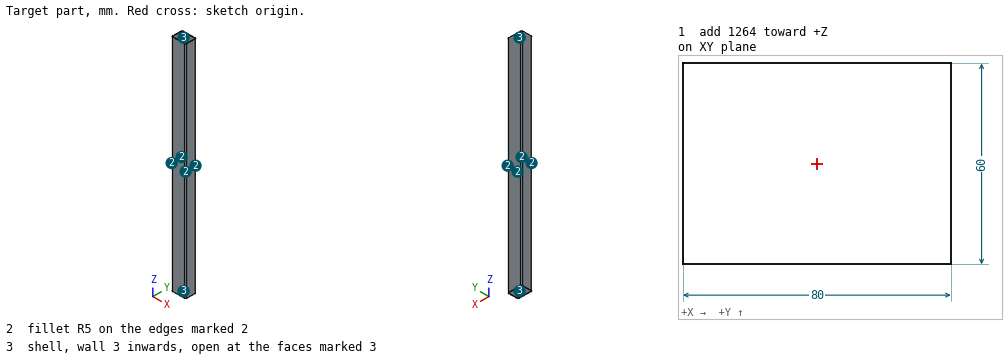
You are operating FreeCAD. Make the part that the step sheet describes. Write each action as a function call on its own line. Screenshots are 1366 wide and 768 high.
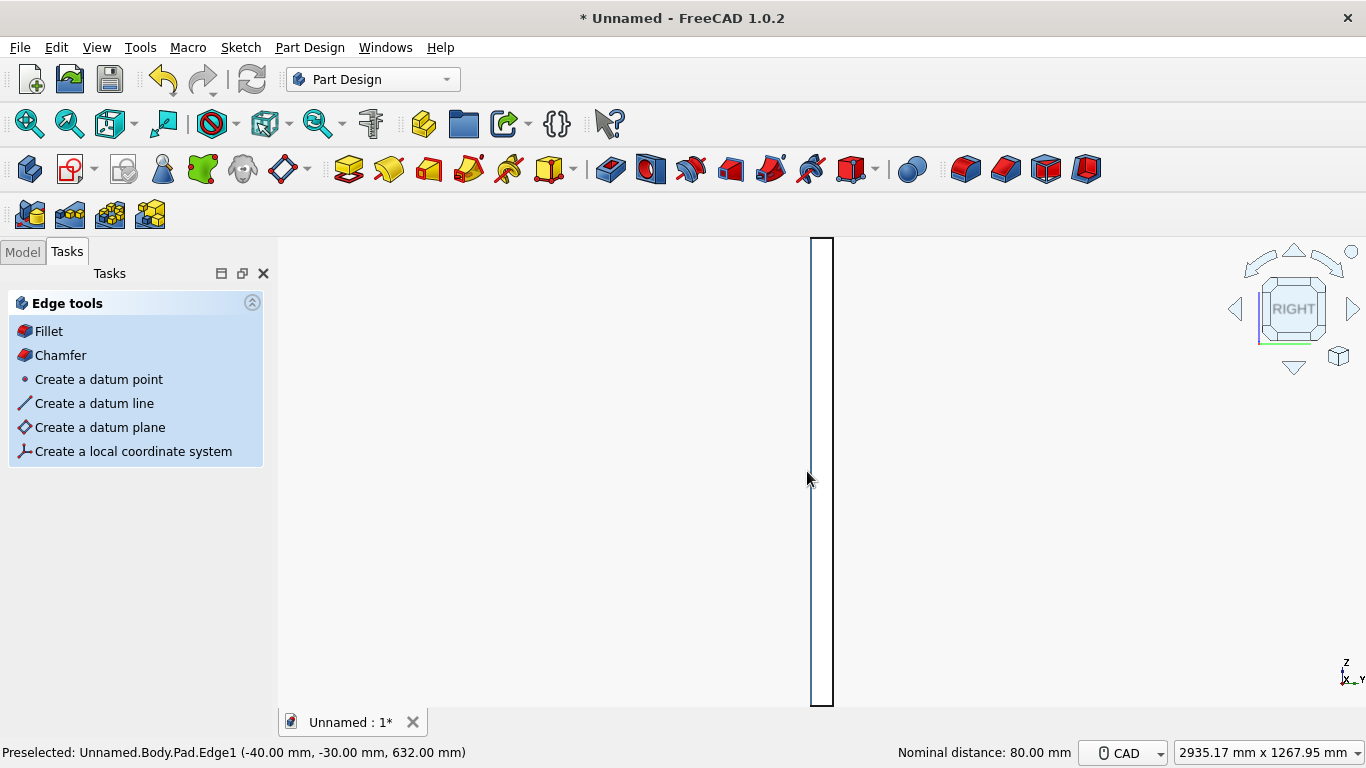
click(833, 471, ctrl)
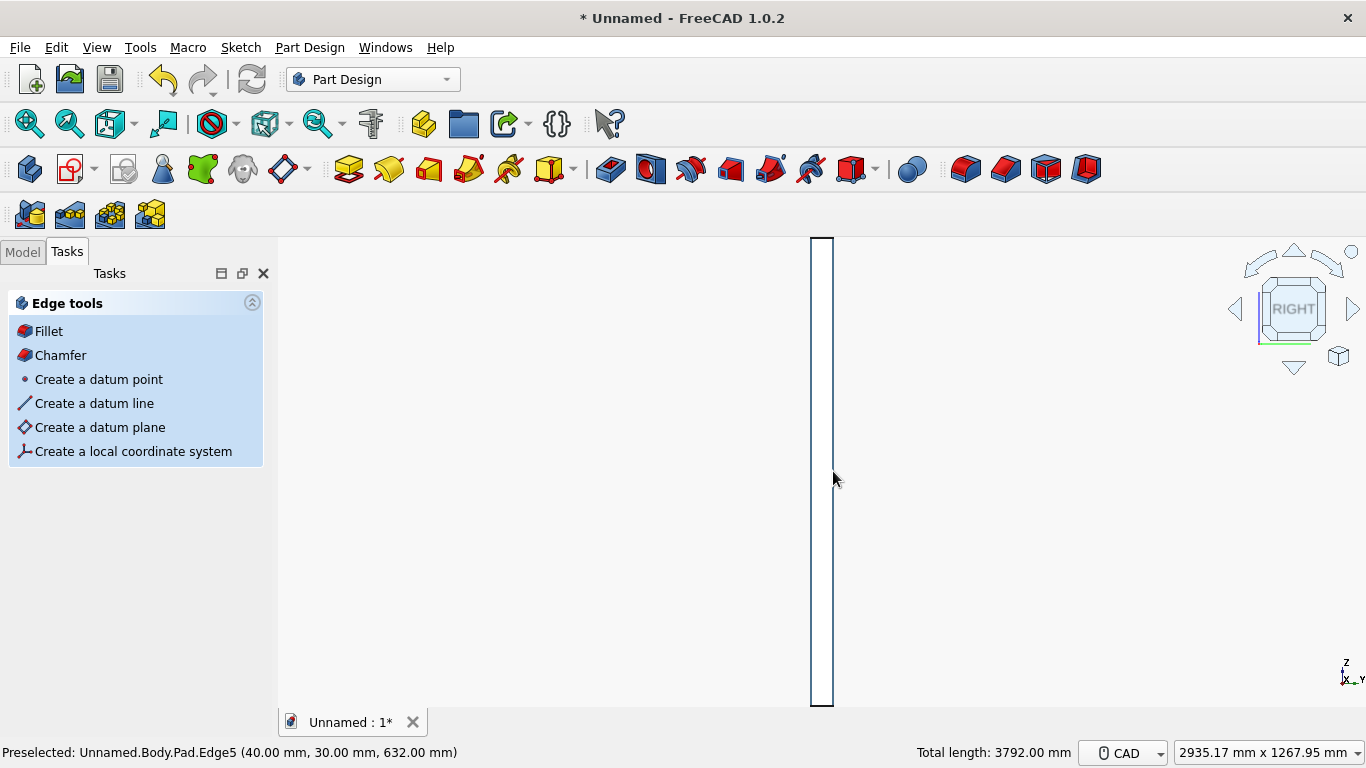
key(5)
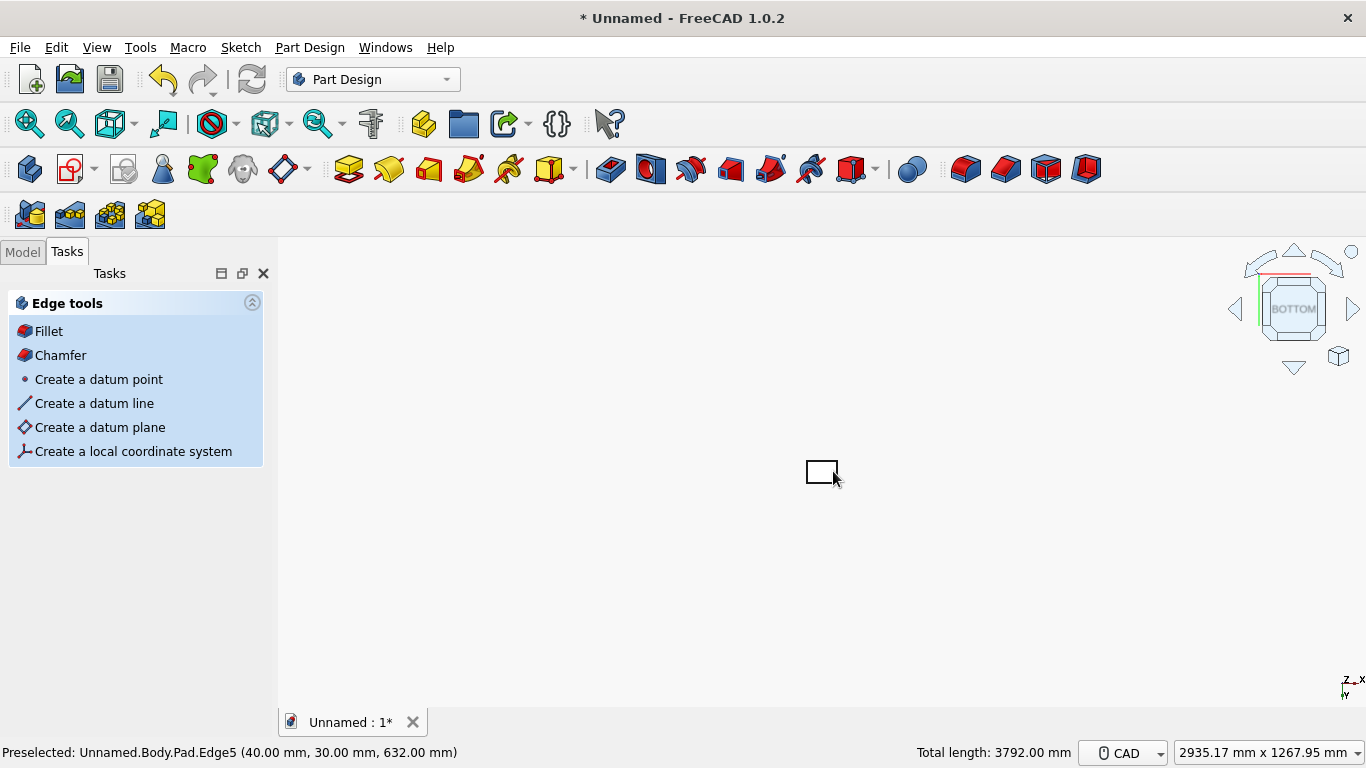
key(v)
key(f)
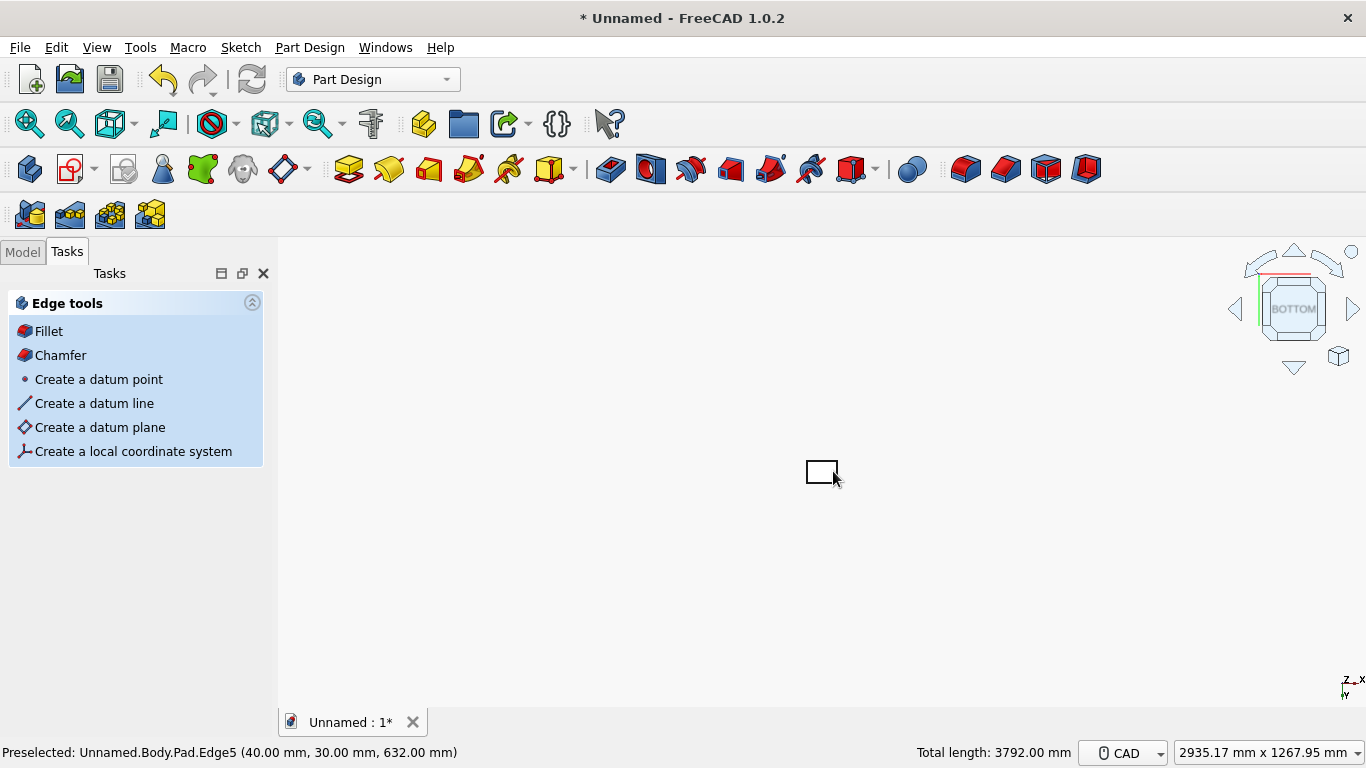
key(4)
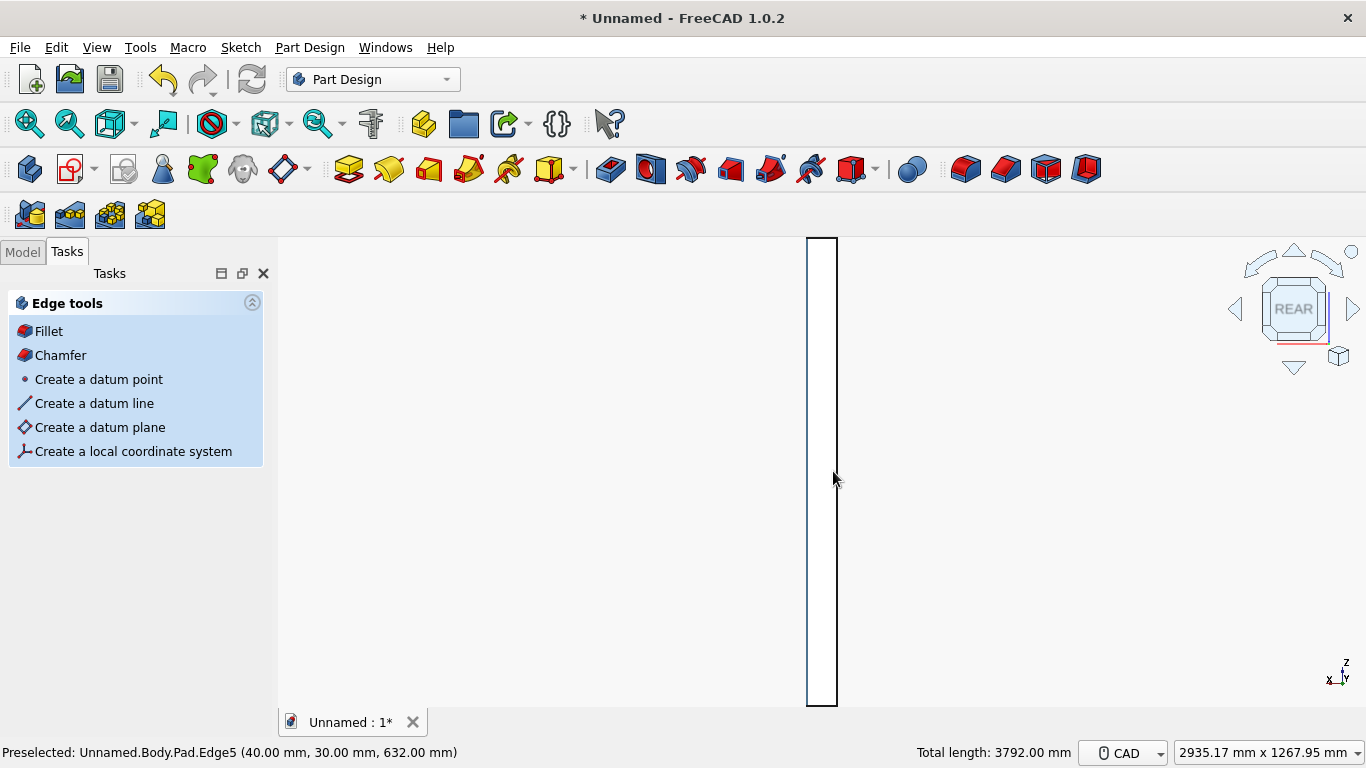
click(837, 471, ctrl)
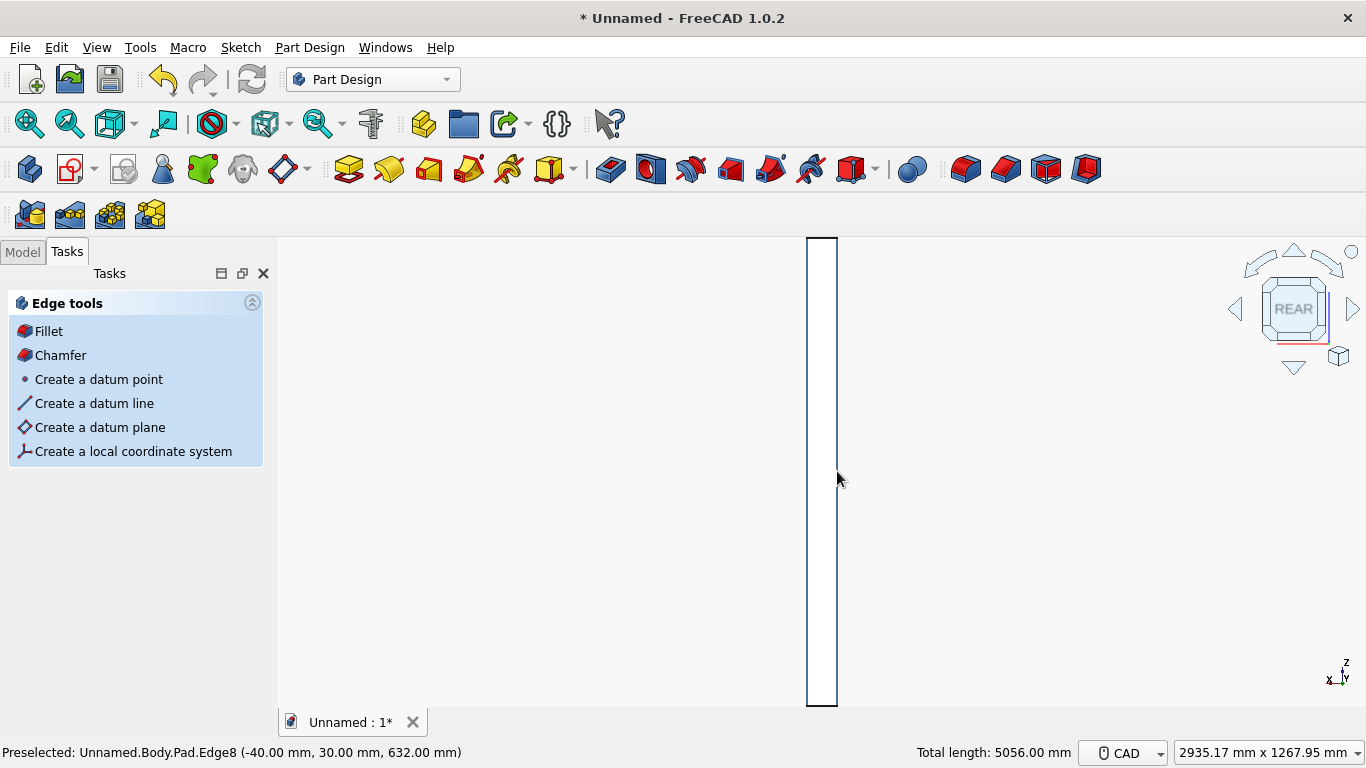
click(966, 170)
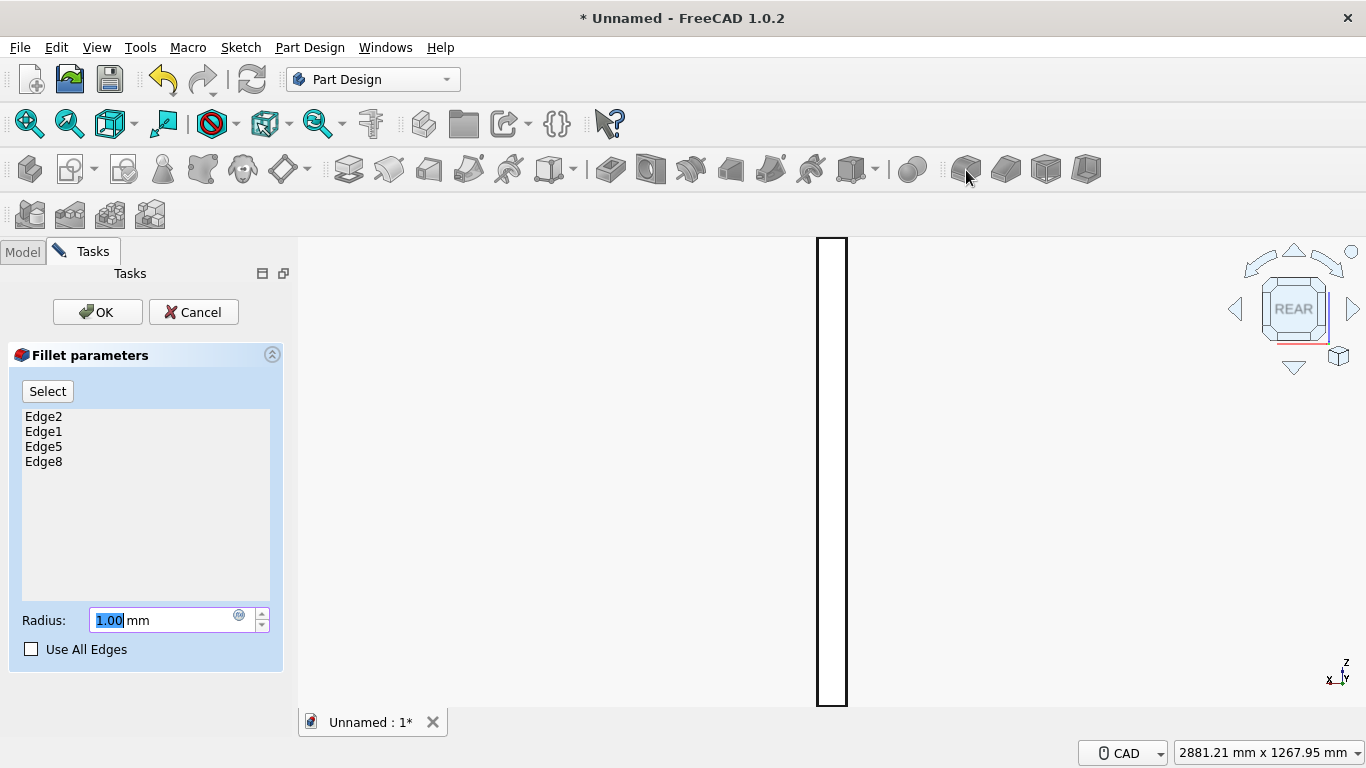
text(5)
key(Tab)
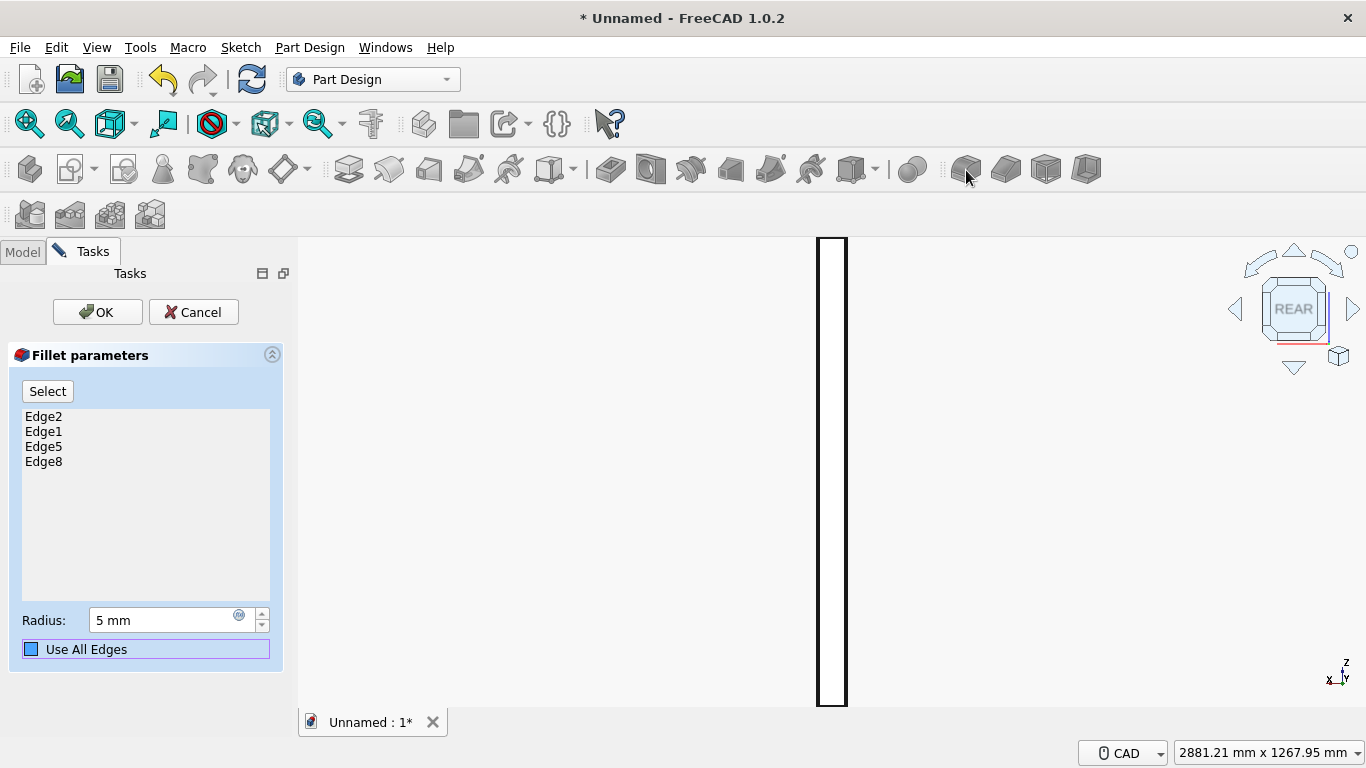
click(98, 312)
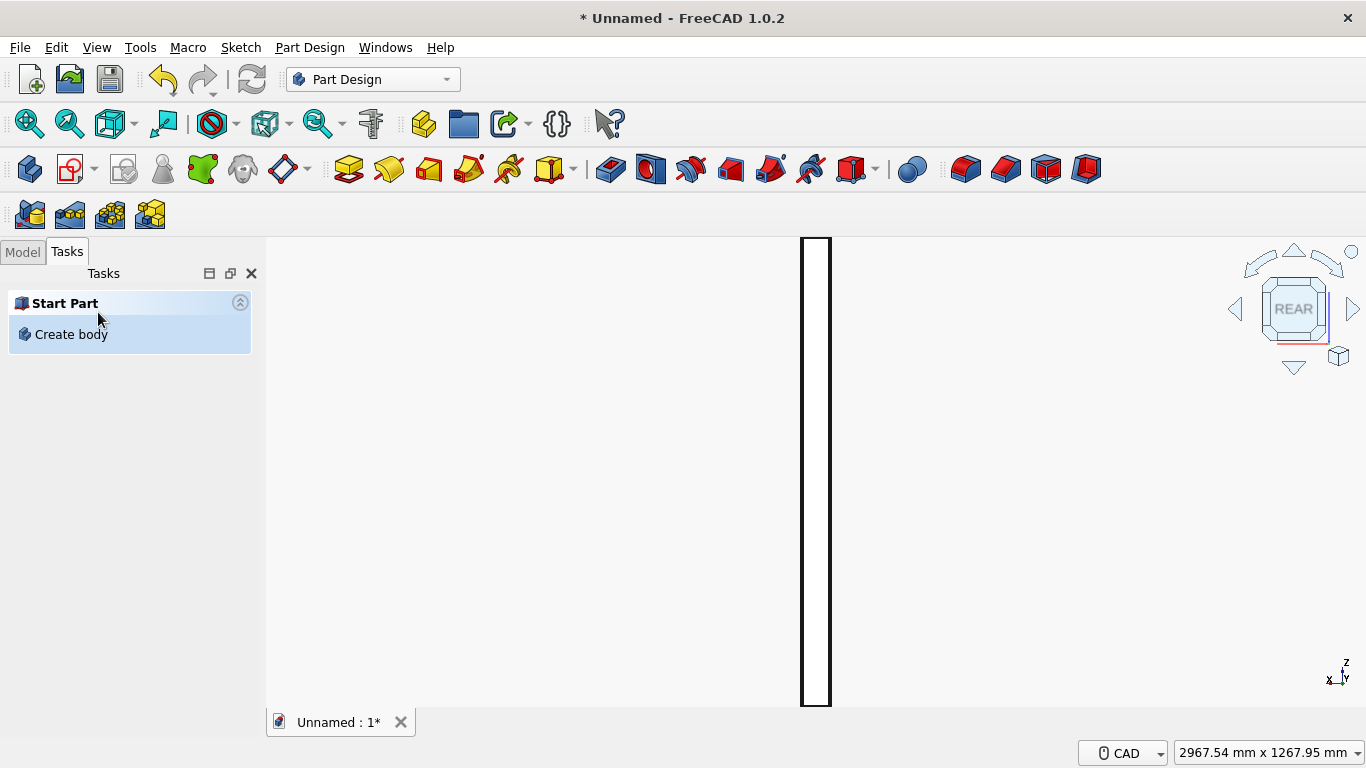
key(0)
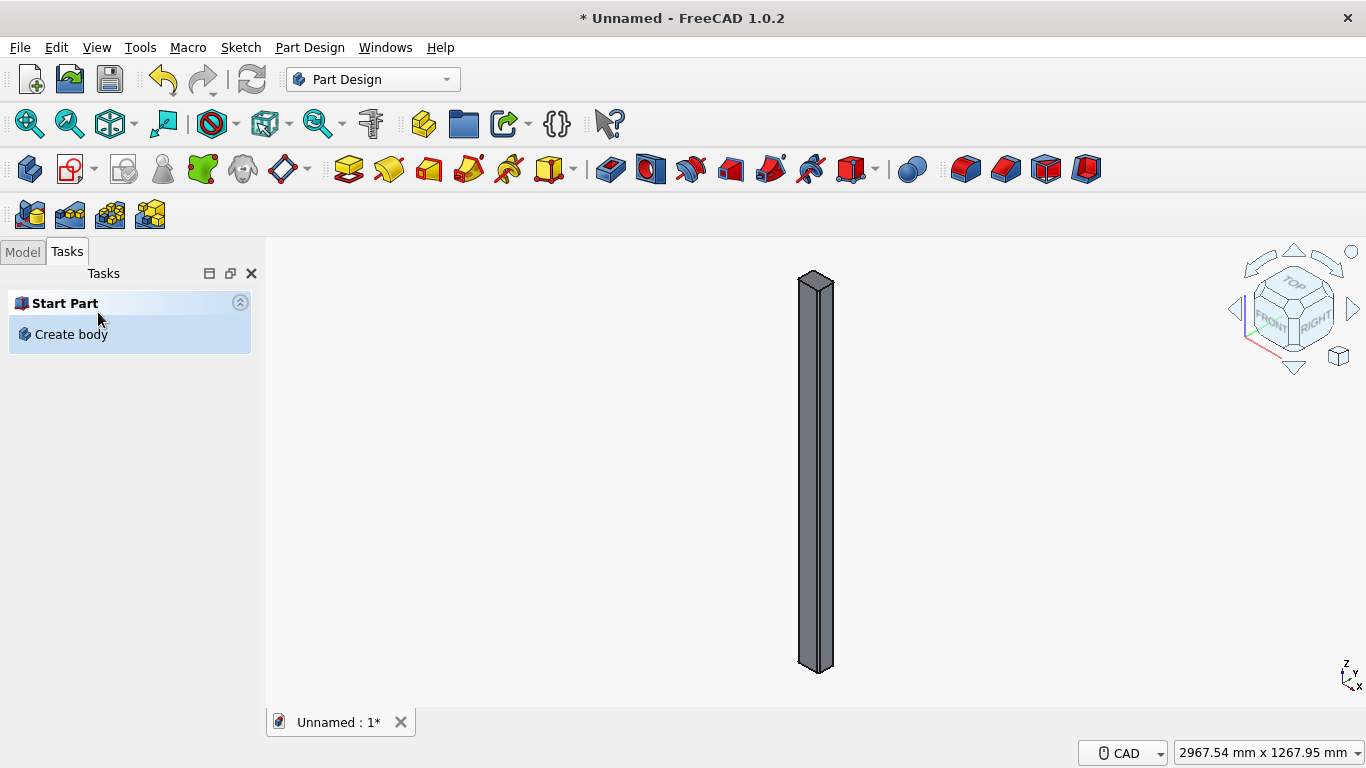
click(818, 278)